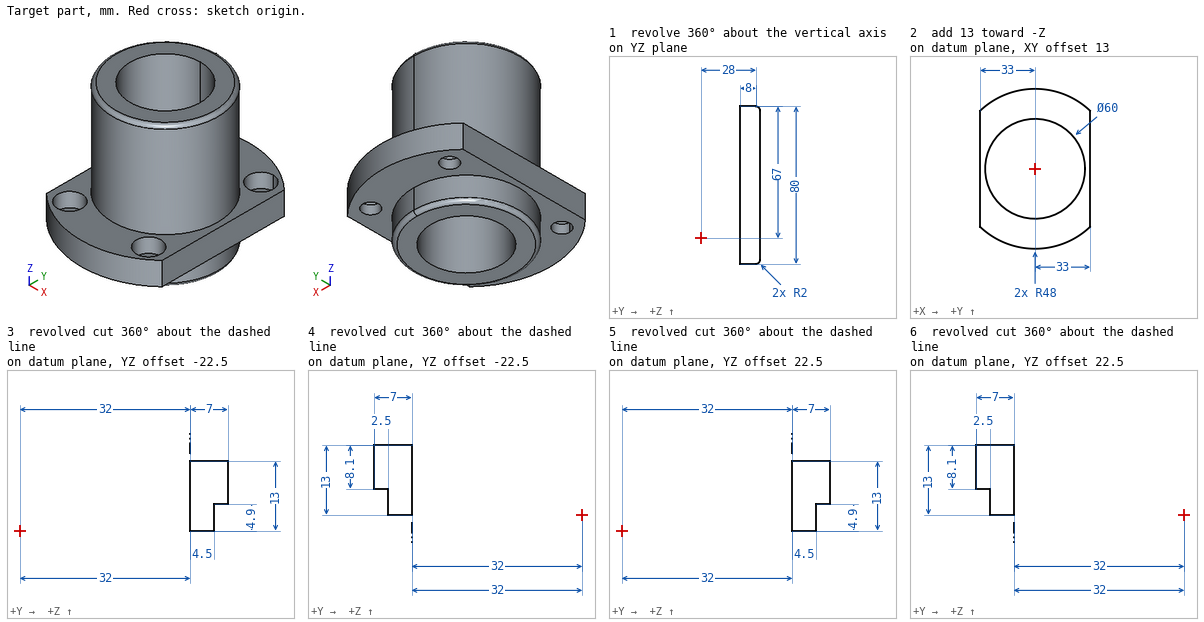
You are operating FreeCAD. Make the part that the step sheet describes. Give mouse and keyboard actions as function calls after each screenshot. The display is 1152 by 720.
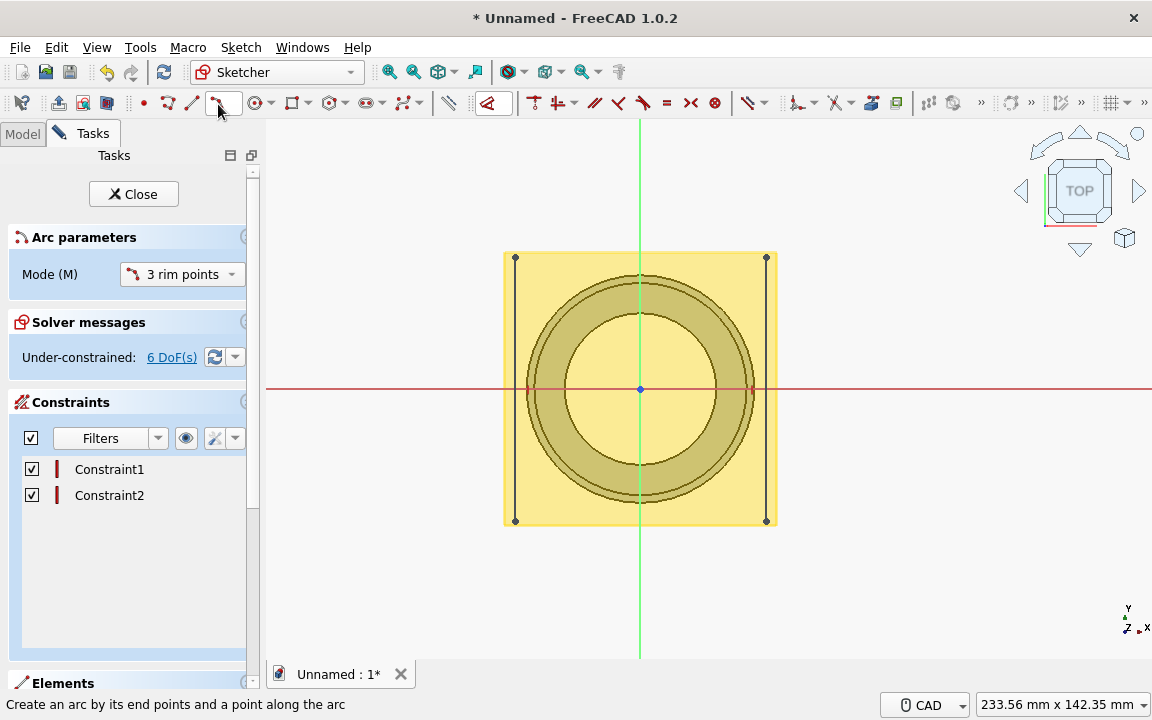
click(515, 522)
click(766, 522)
click(613, 569)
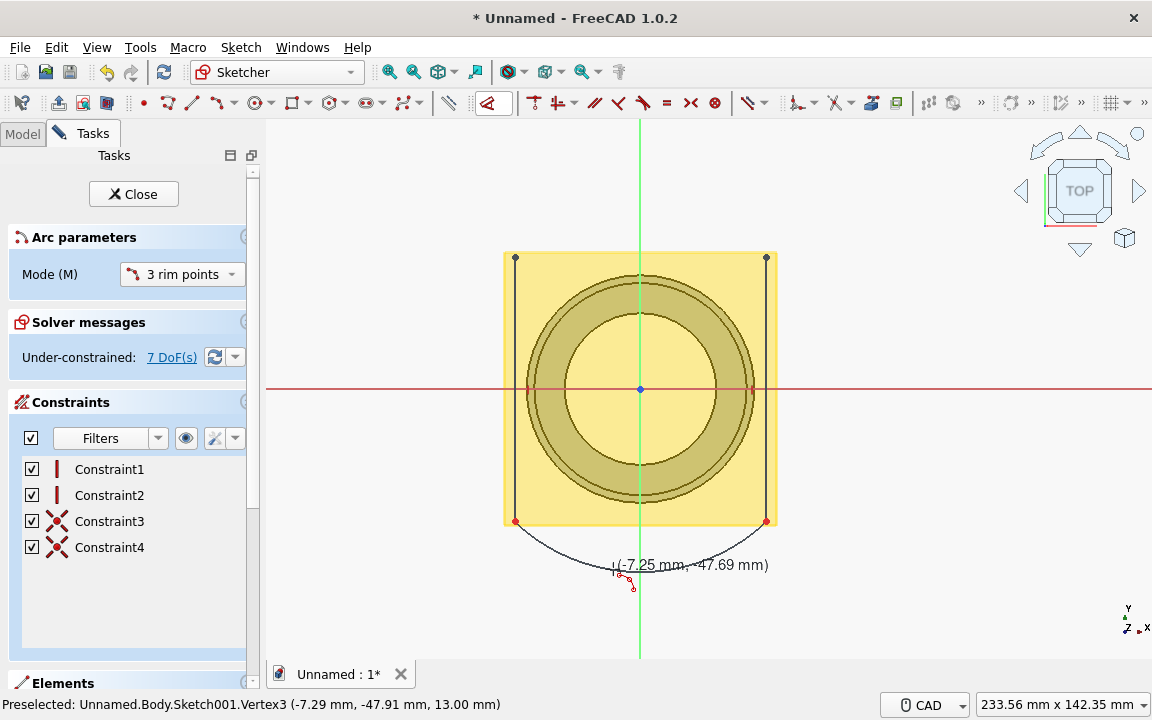
click(766, 258)
click(515, 258)
click(668, 209)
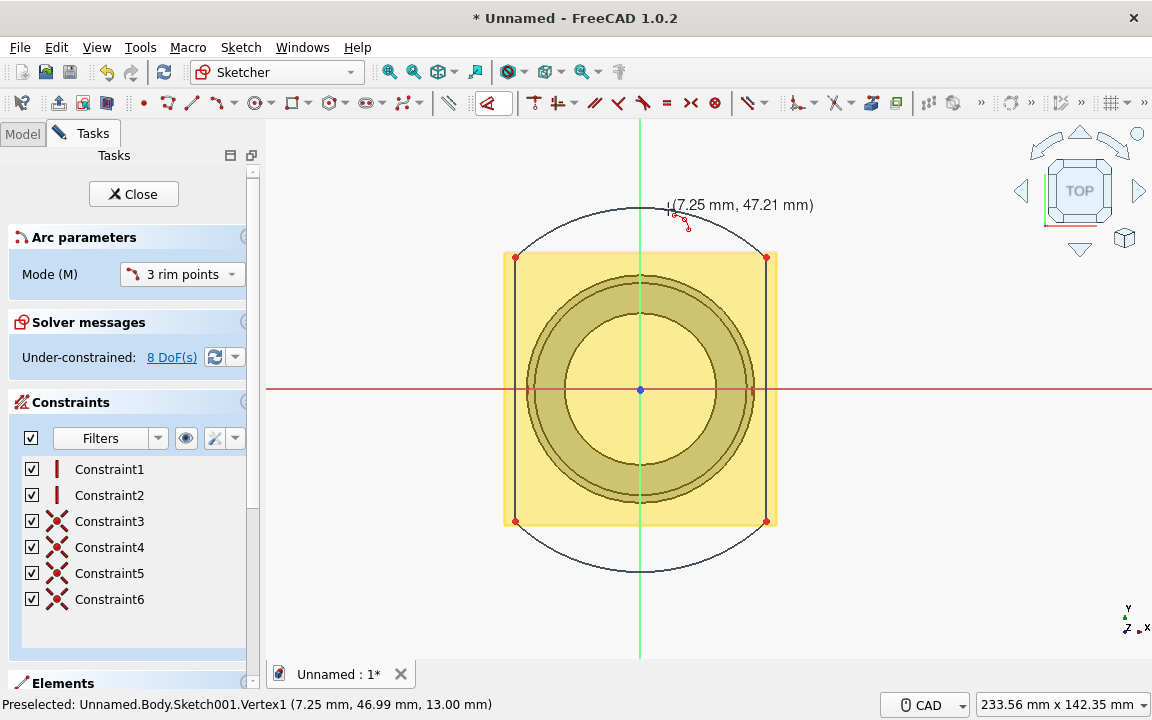
click(256, 104)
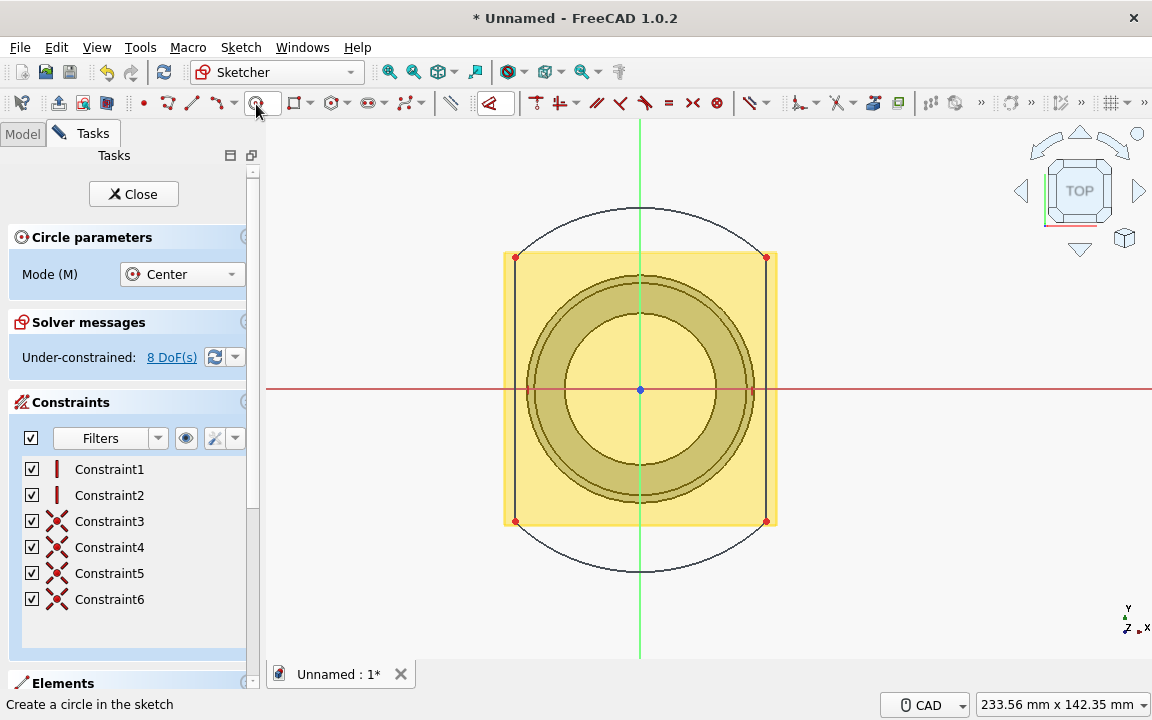
click(640, 389)
move(721, 309)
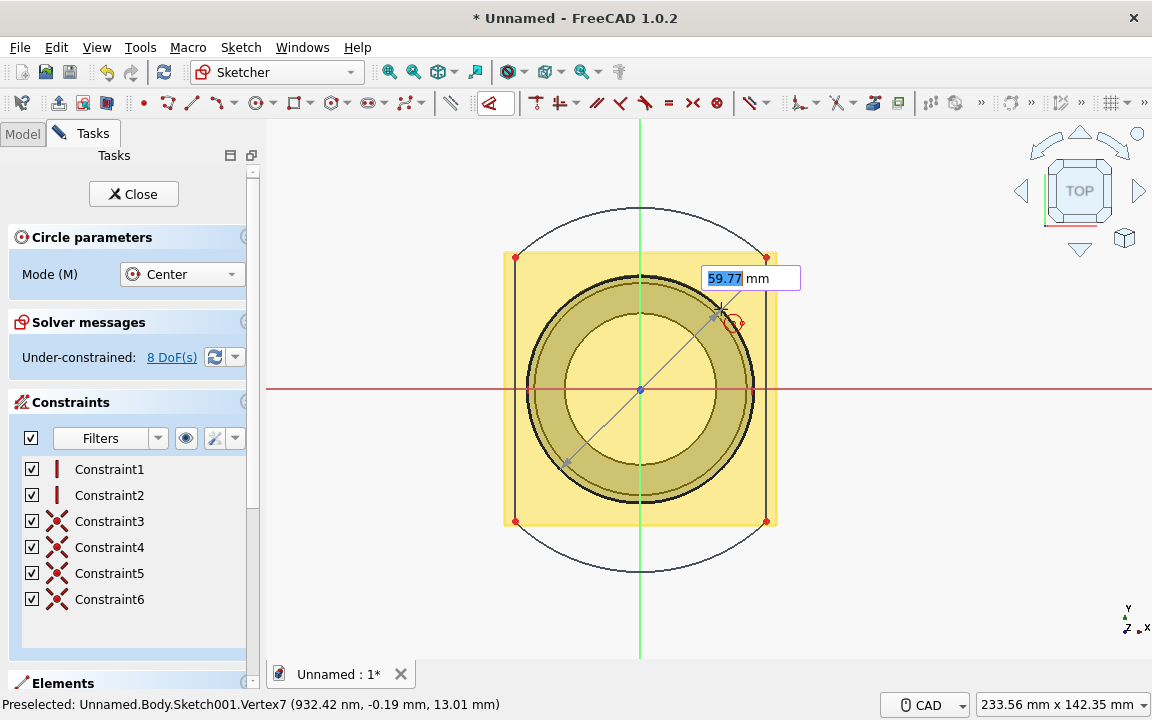
text(60)
key(Return)
key(Escape)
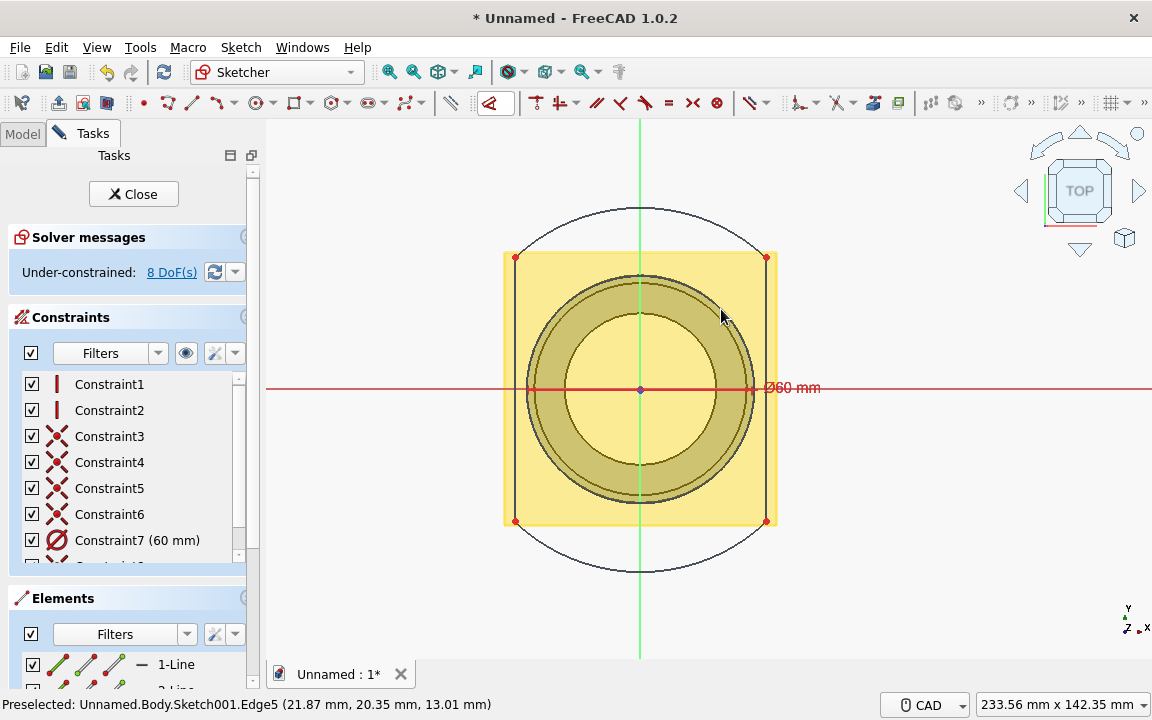
click(721, 309)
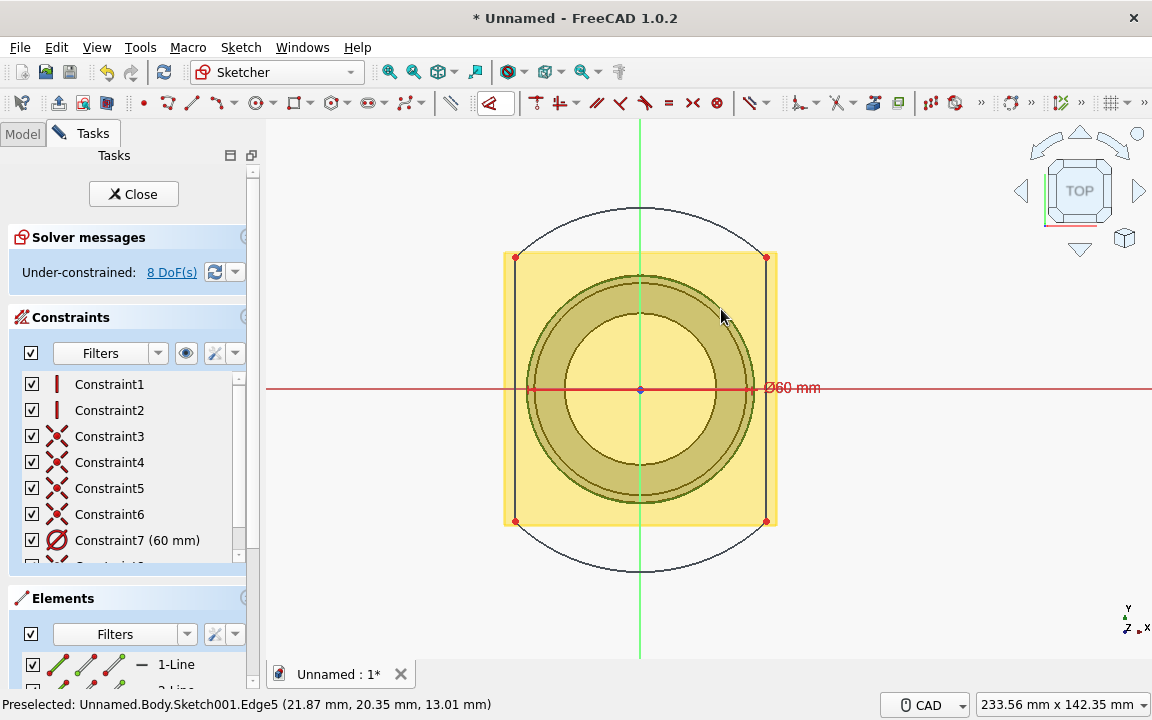
click(695, 216)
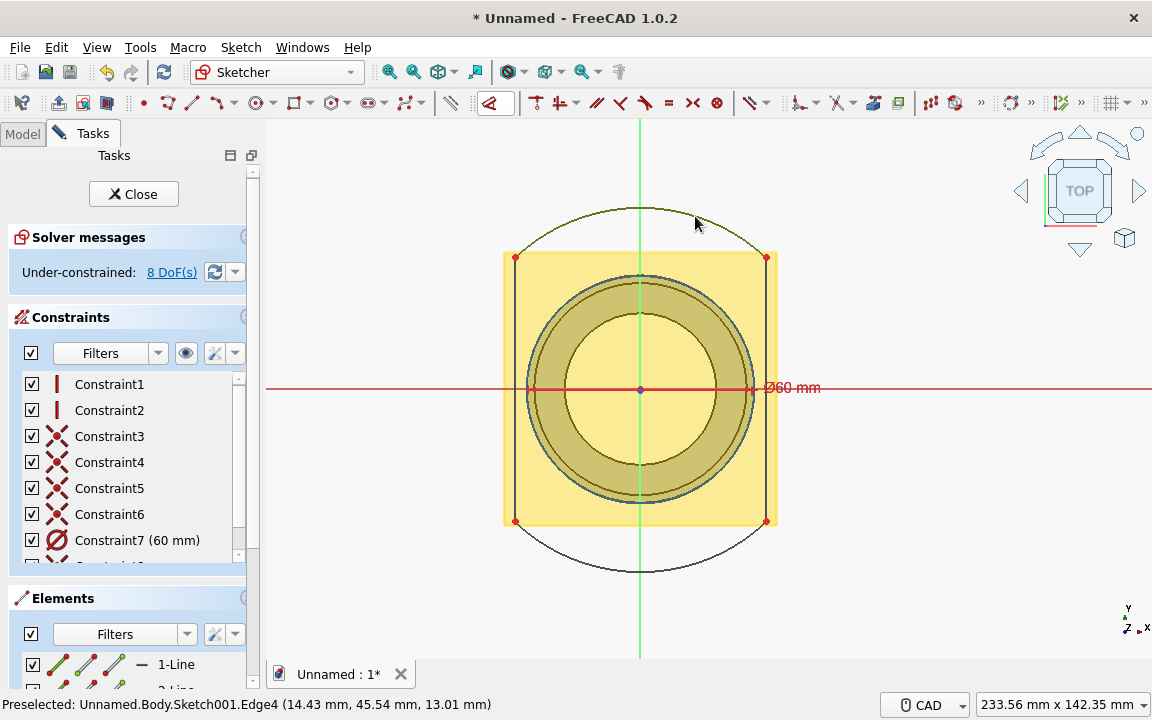
click(536, 104)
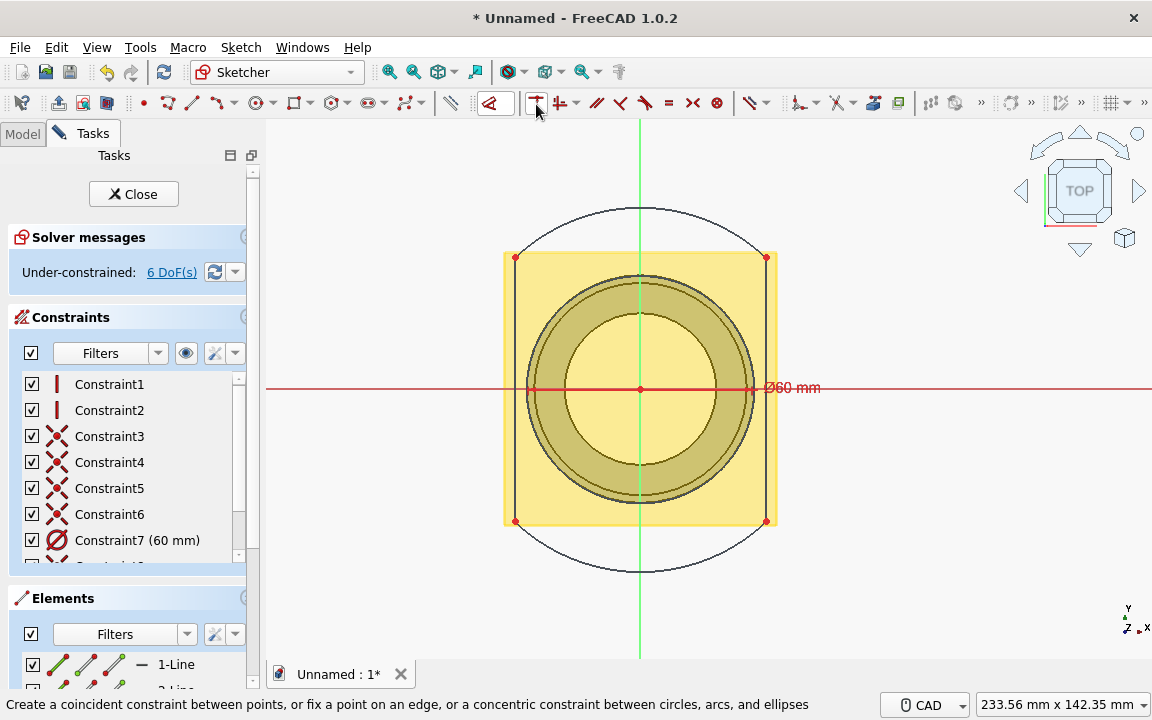
drag(630, 379, 651, 400)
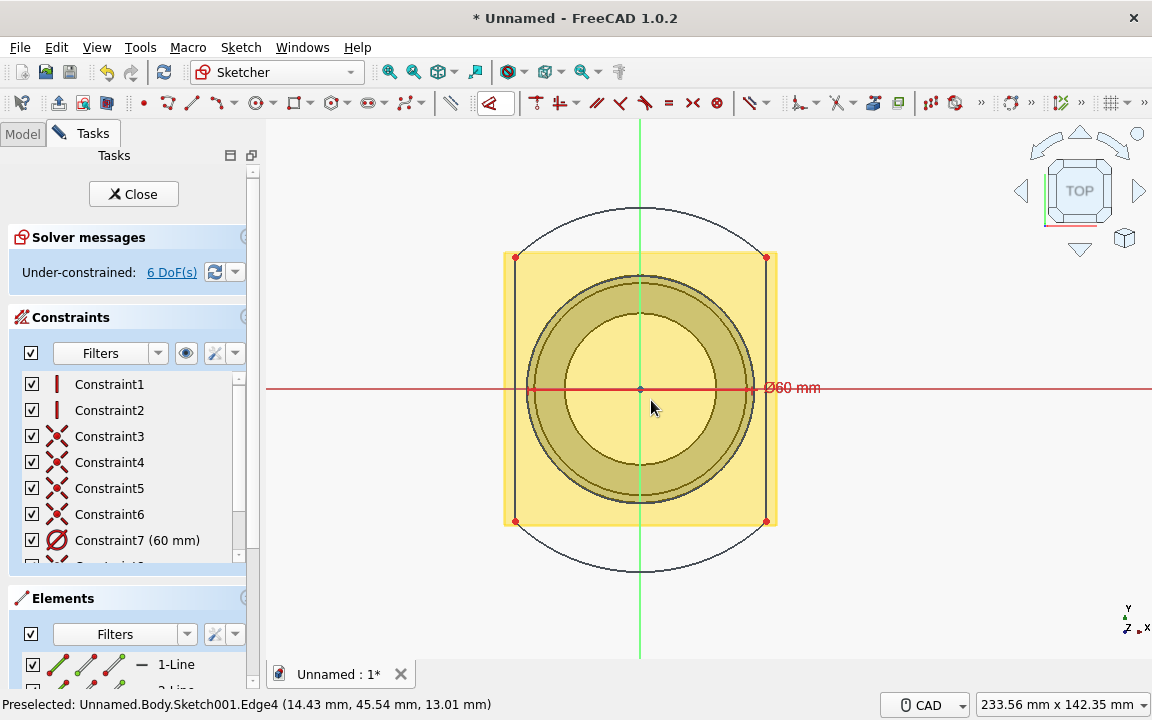
click(536, 104)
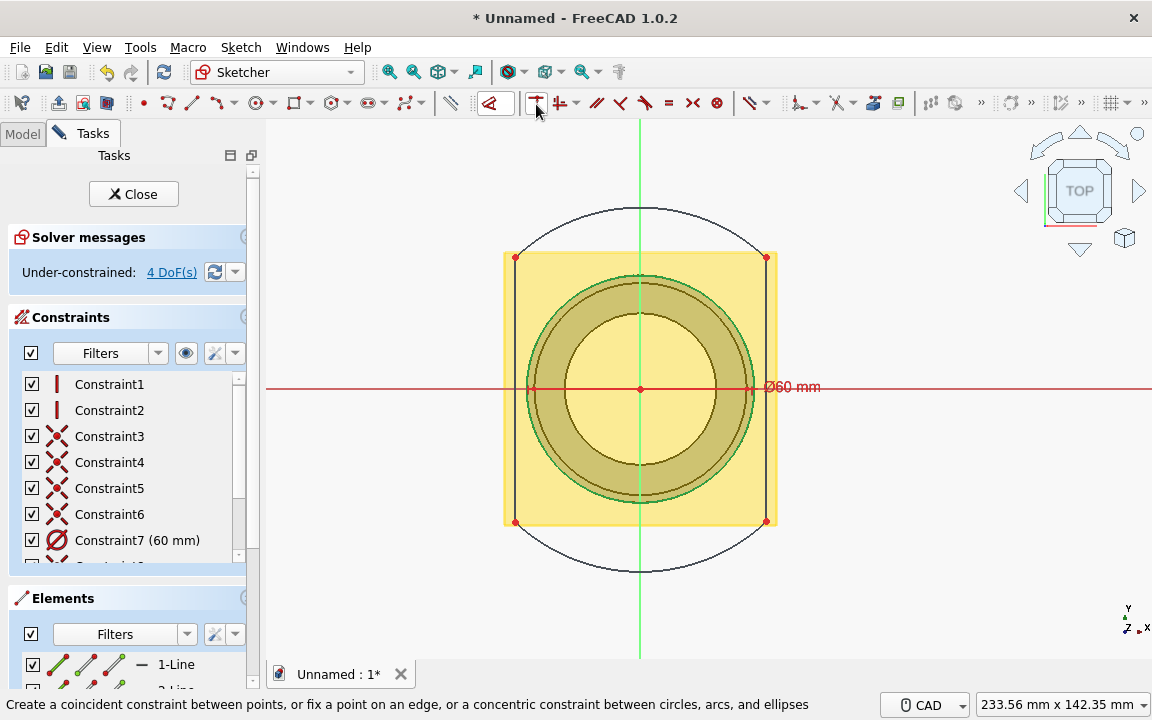
click(586, 564)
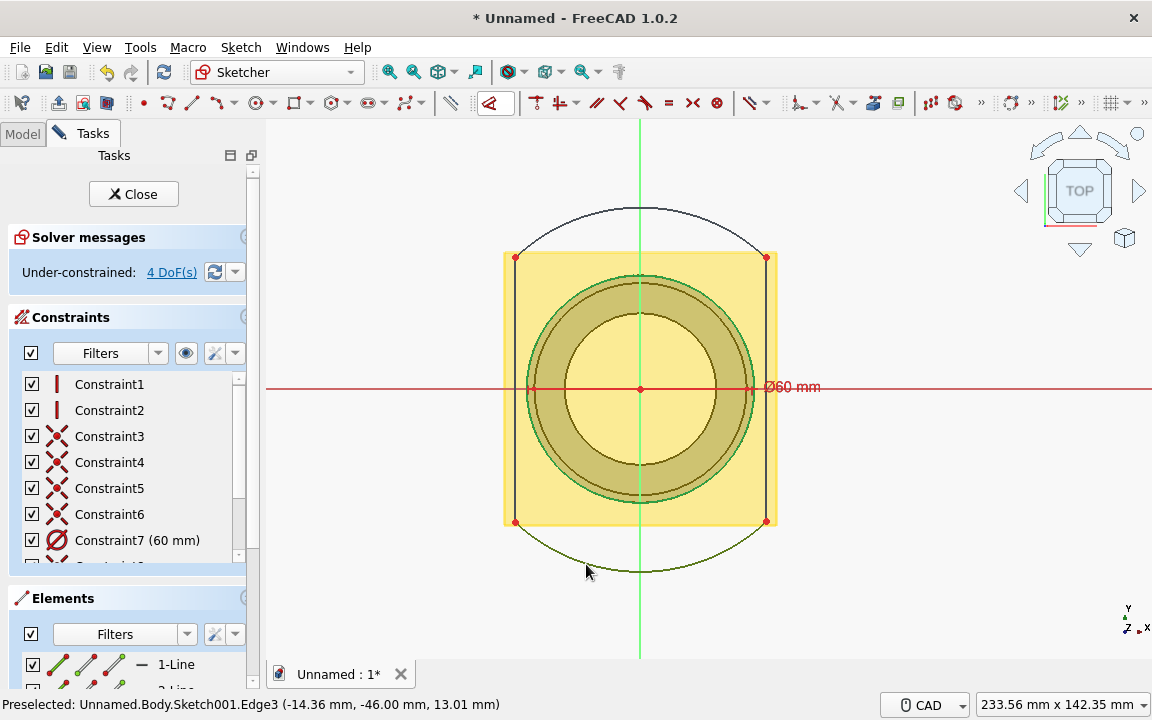
click(695, 216)